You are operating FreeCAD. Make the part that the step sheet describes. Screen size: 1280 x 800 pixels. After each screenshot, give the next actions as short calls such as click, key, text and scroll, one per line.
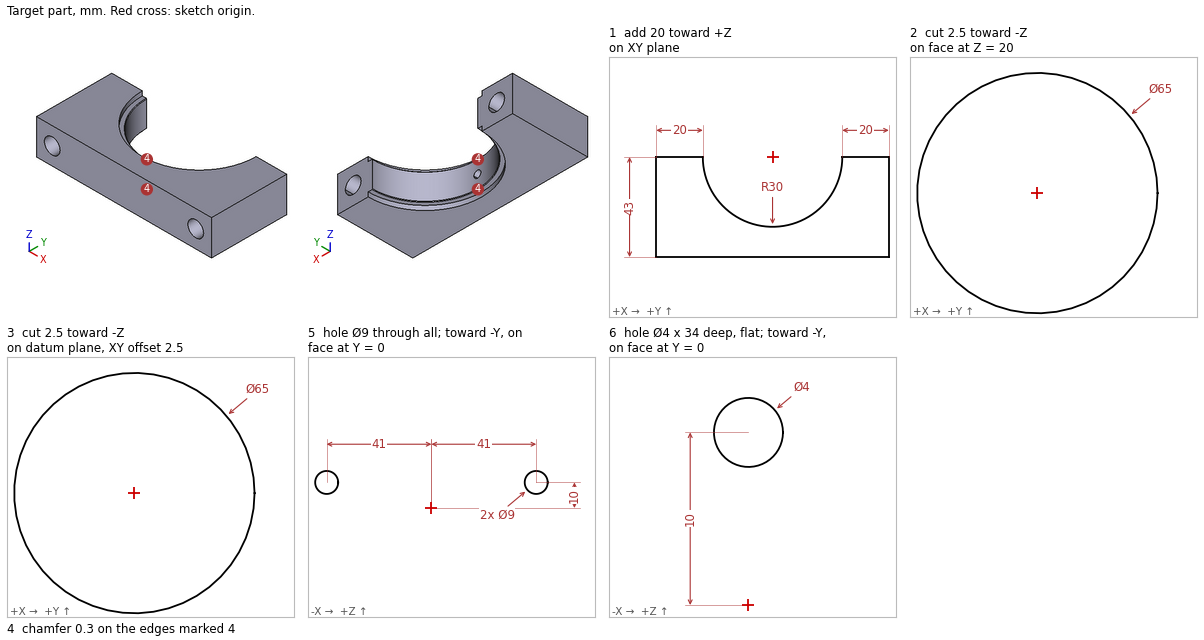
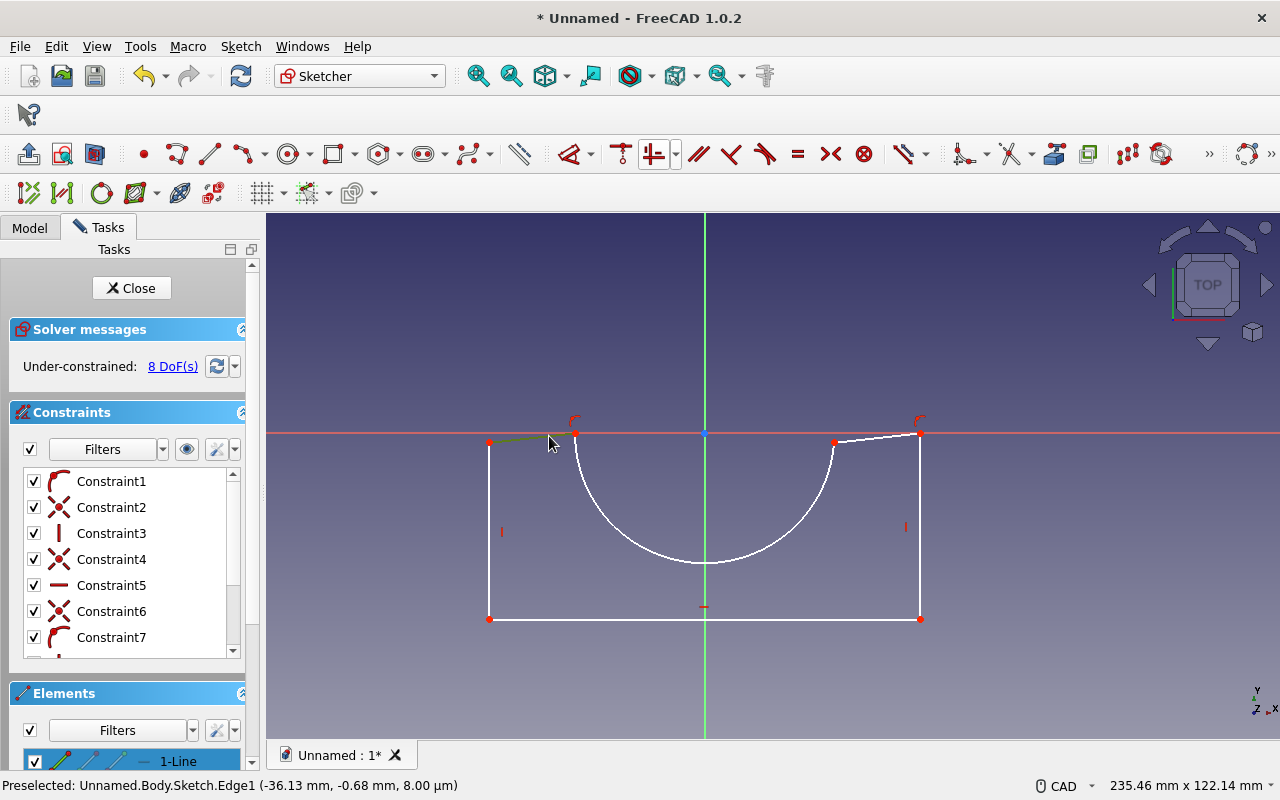
click(676, 154)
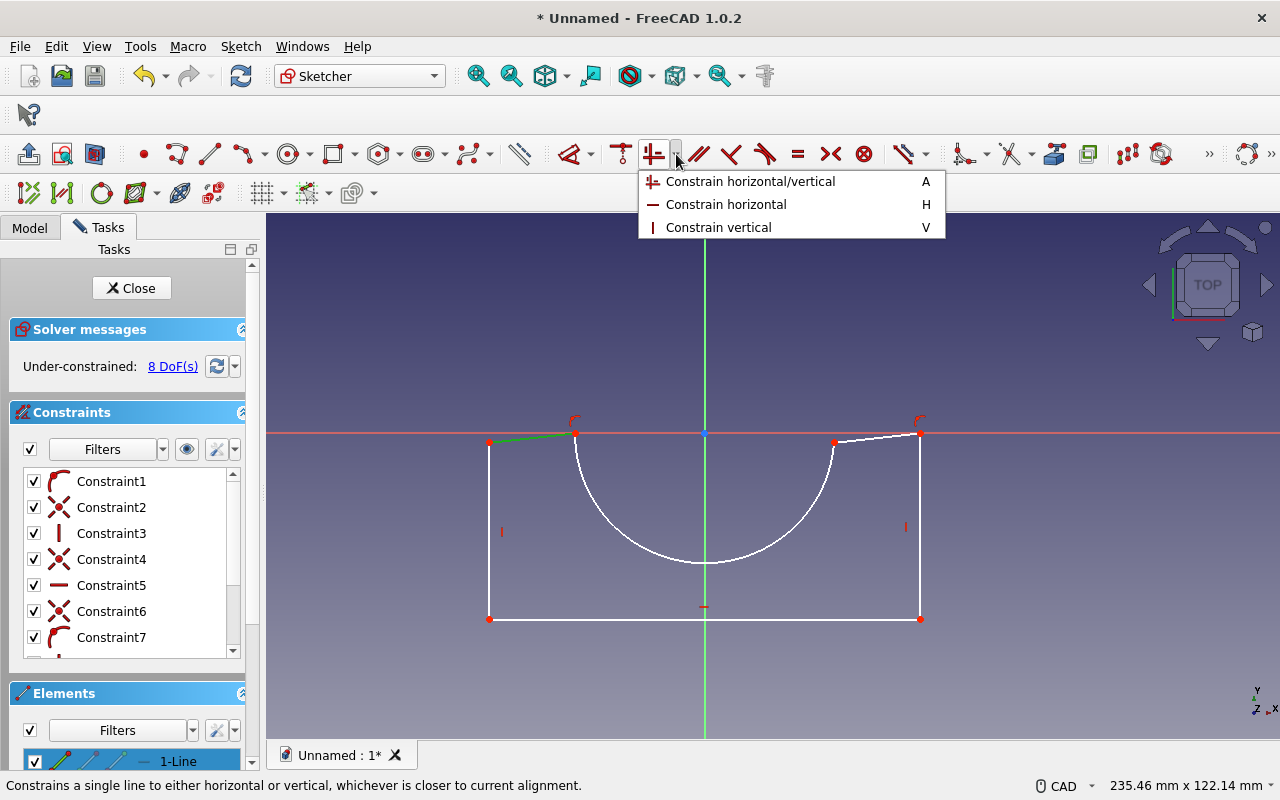
click(792, 204)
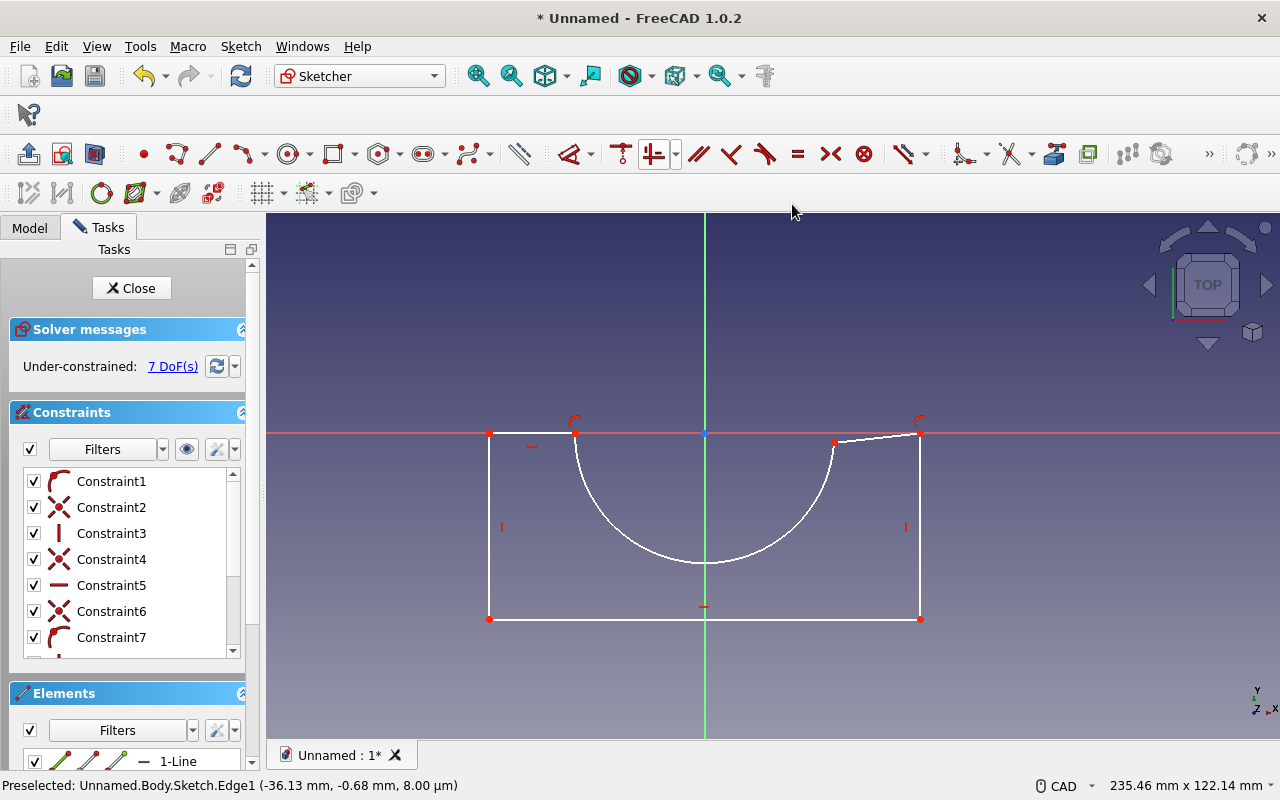
click(894, 436)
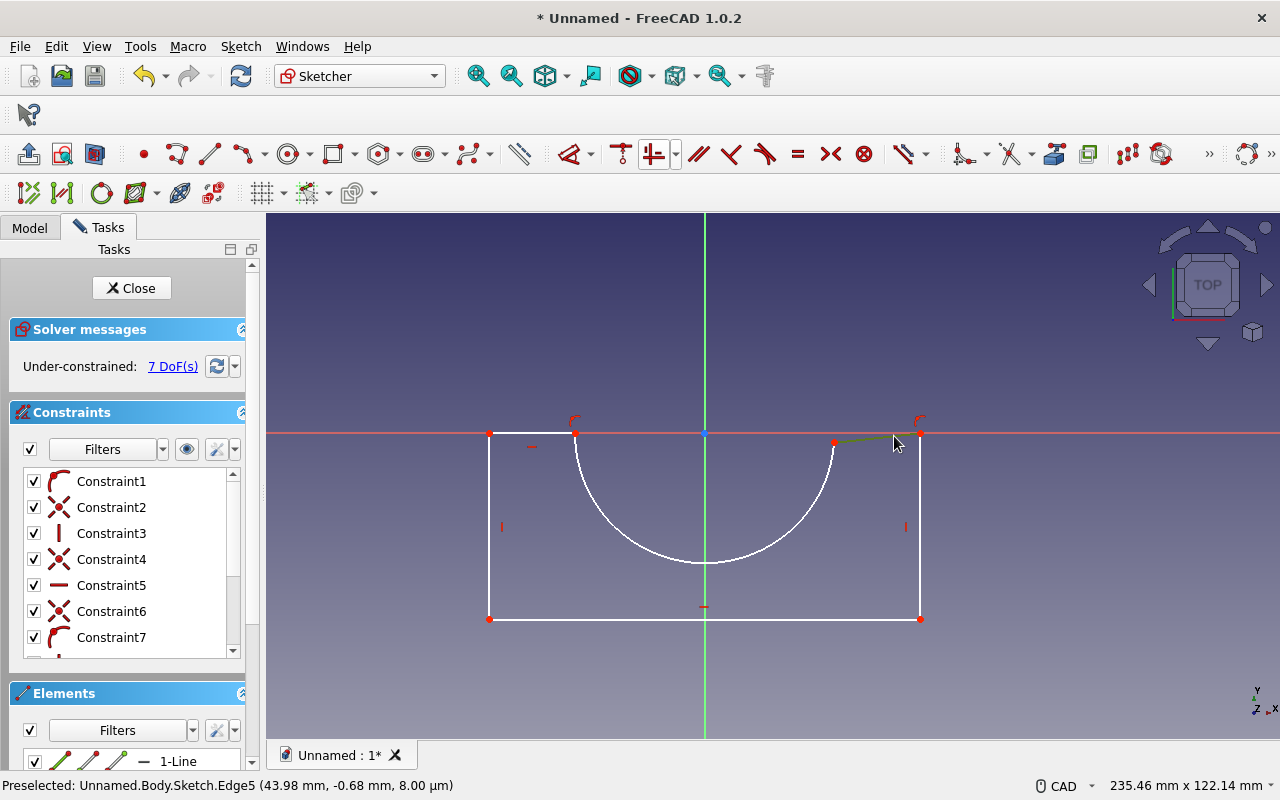
click(676, 154)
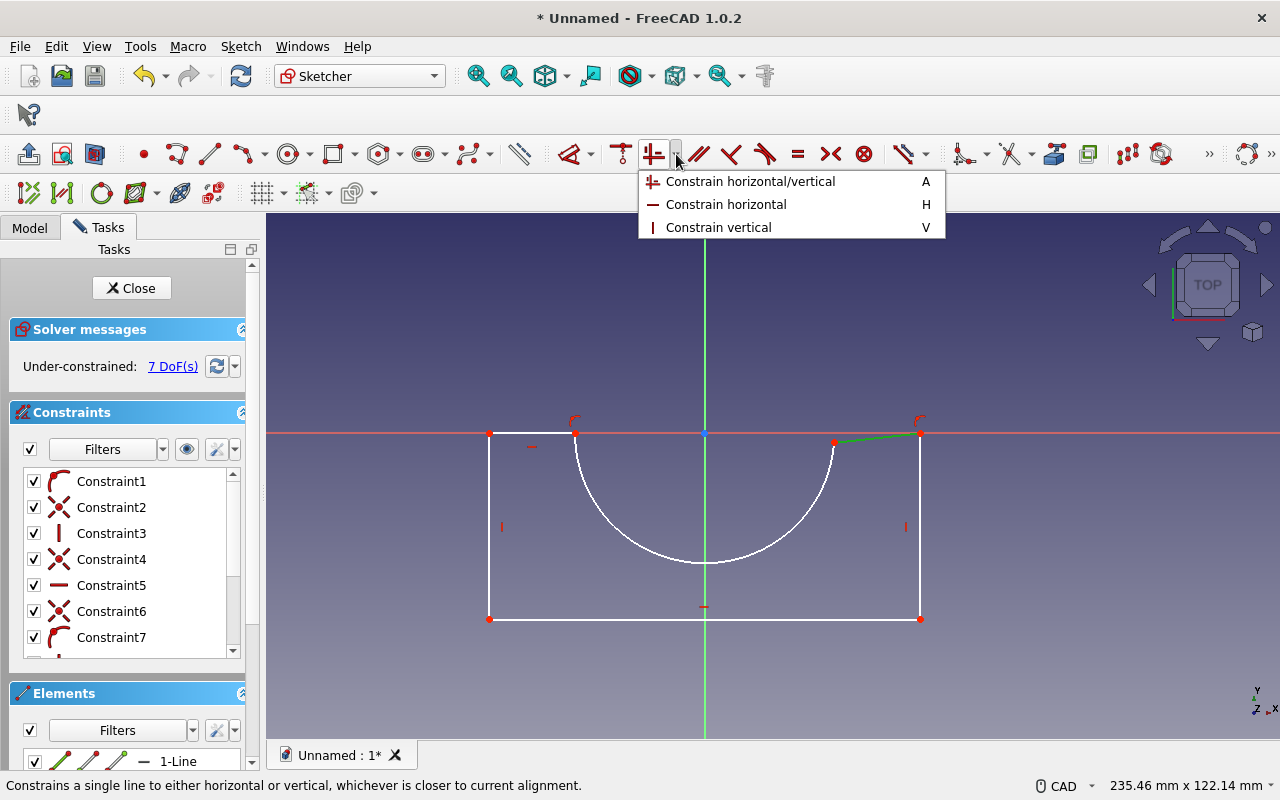
click(792, 204)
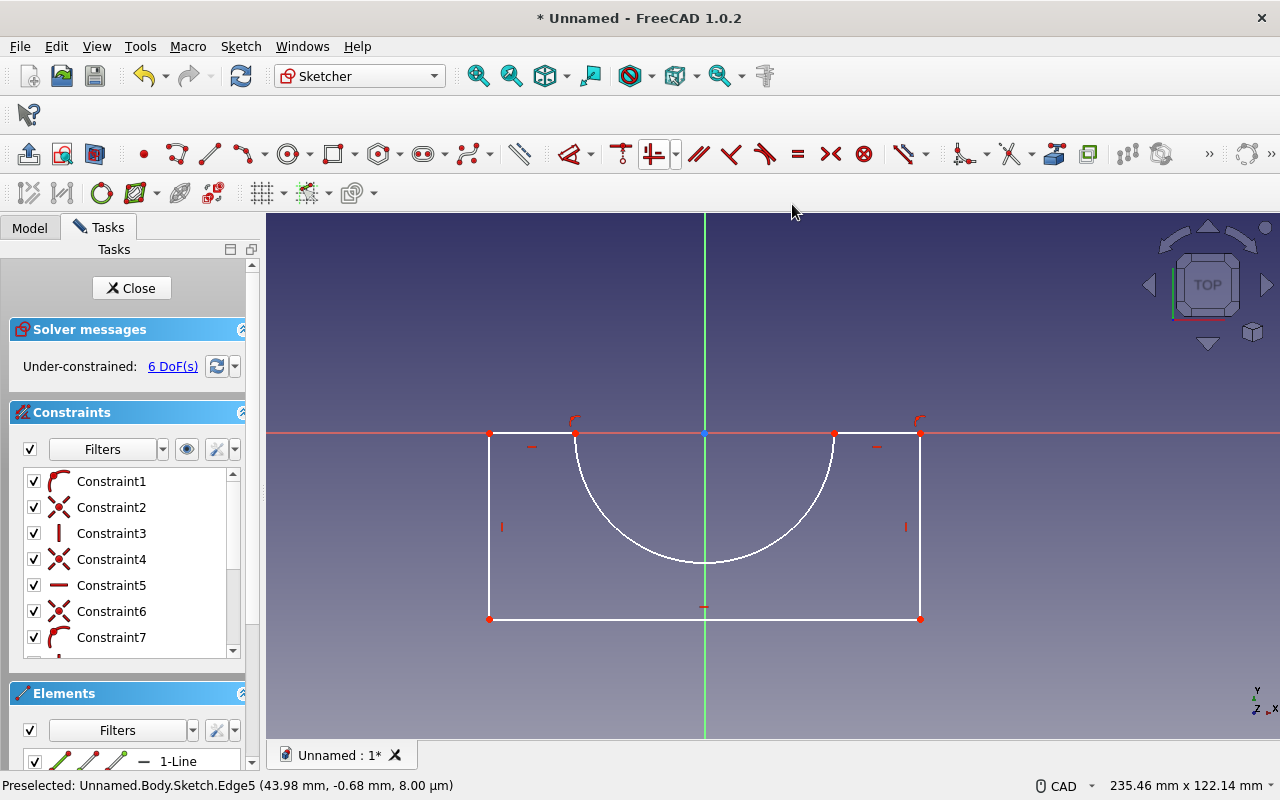
drag(695, 423, 715, 444)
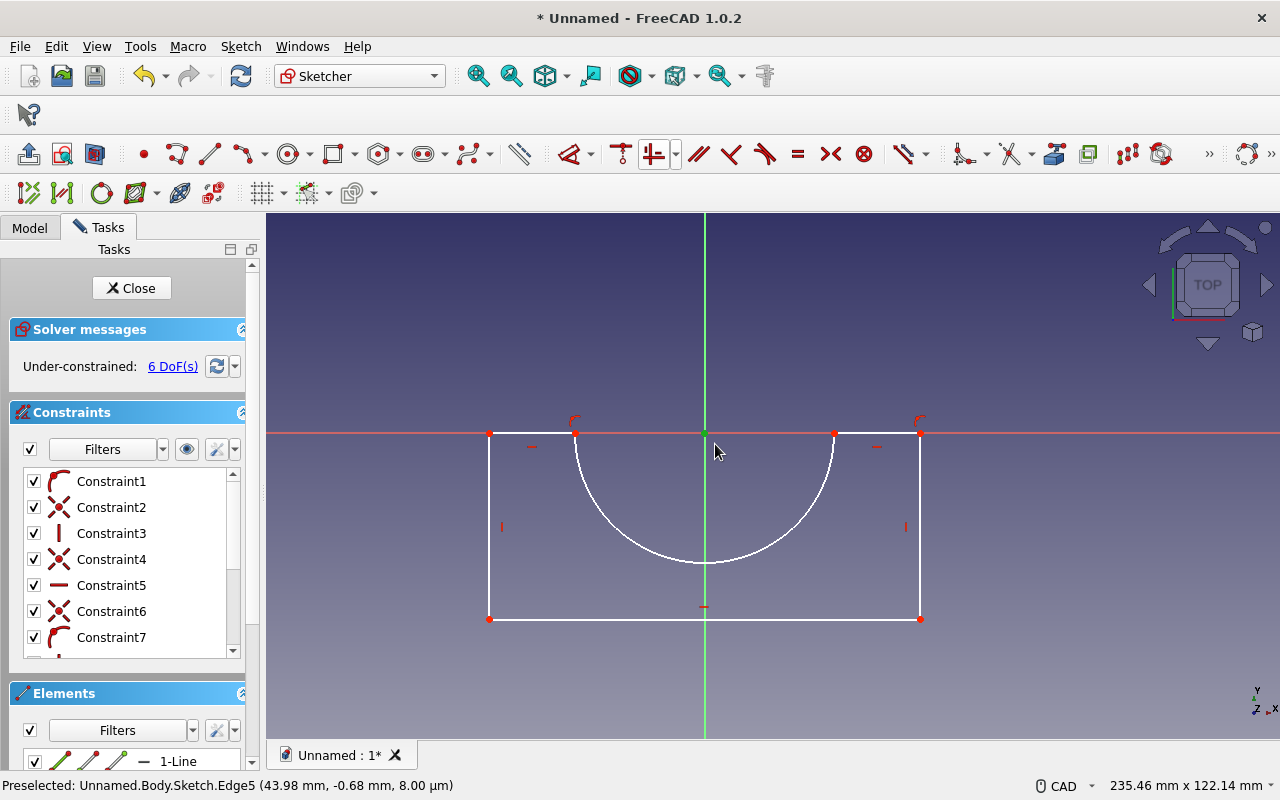
click(621, 154)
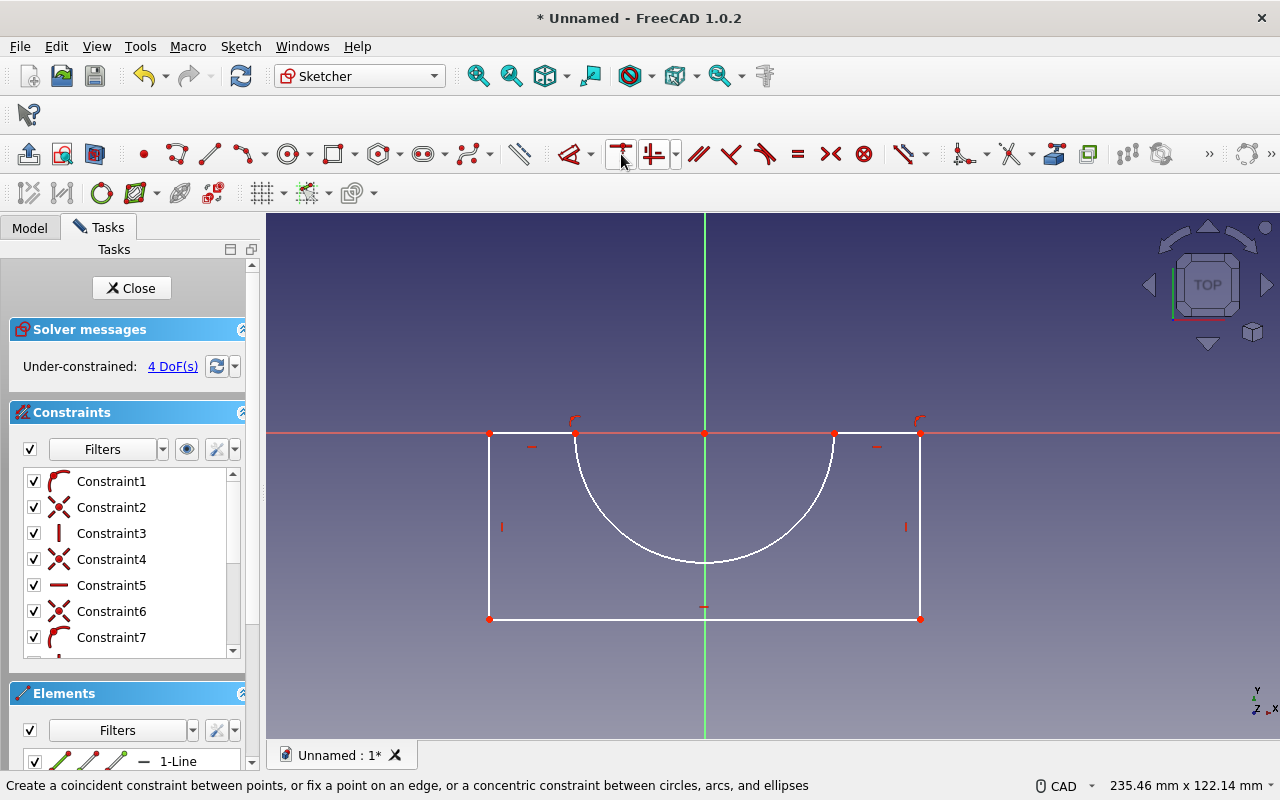
click(568, 154)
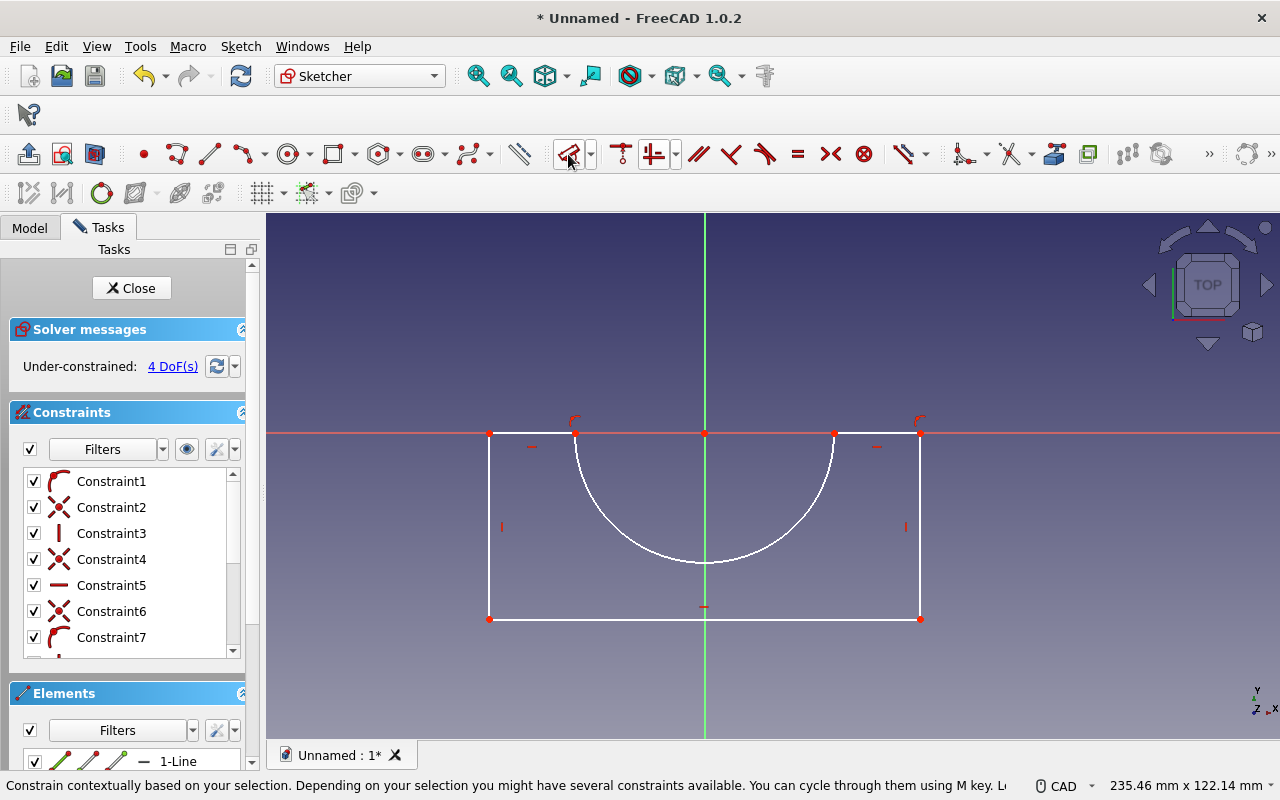
click(628, 538)
click(609, 564)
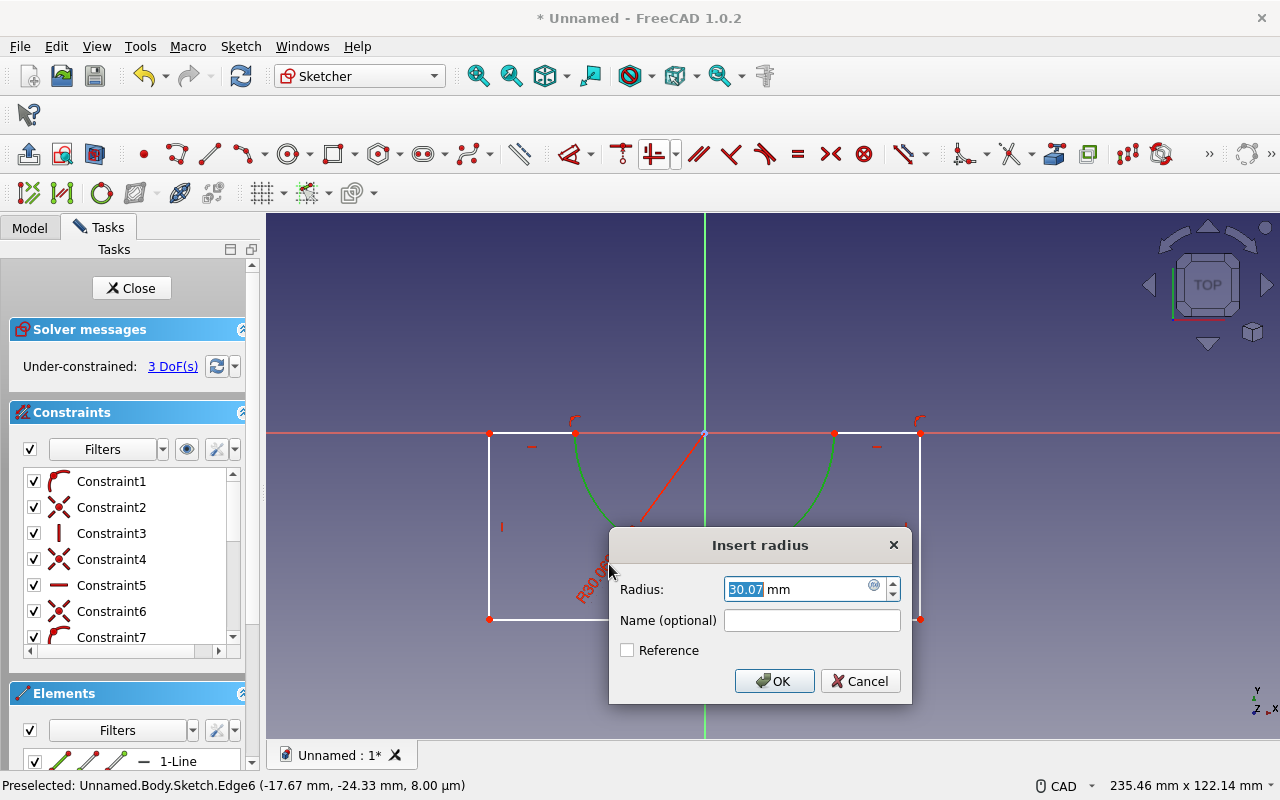
text(30)
key(Return)